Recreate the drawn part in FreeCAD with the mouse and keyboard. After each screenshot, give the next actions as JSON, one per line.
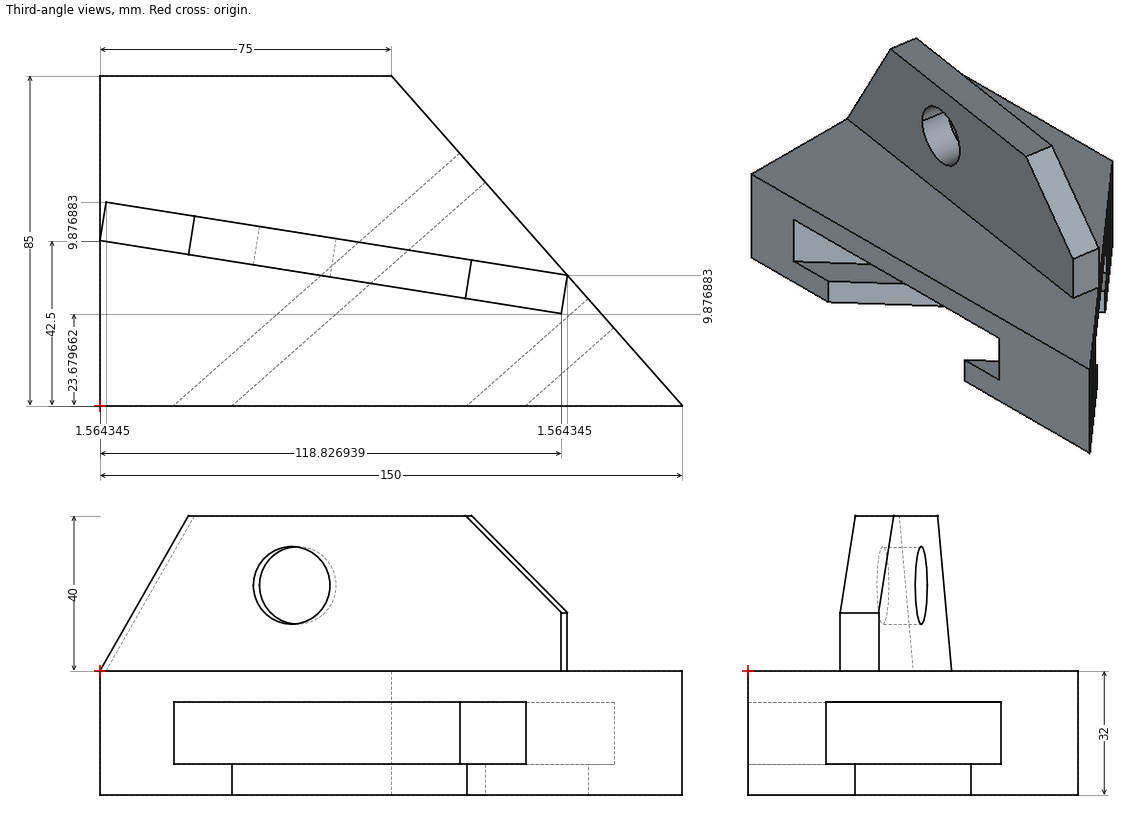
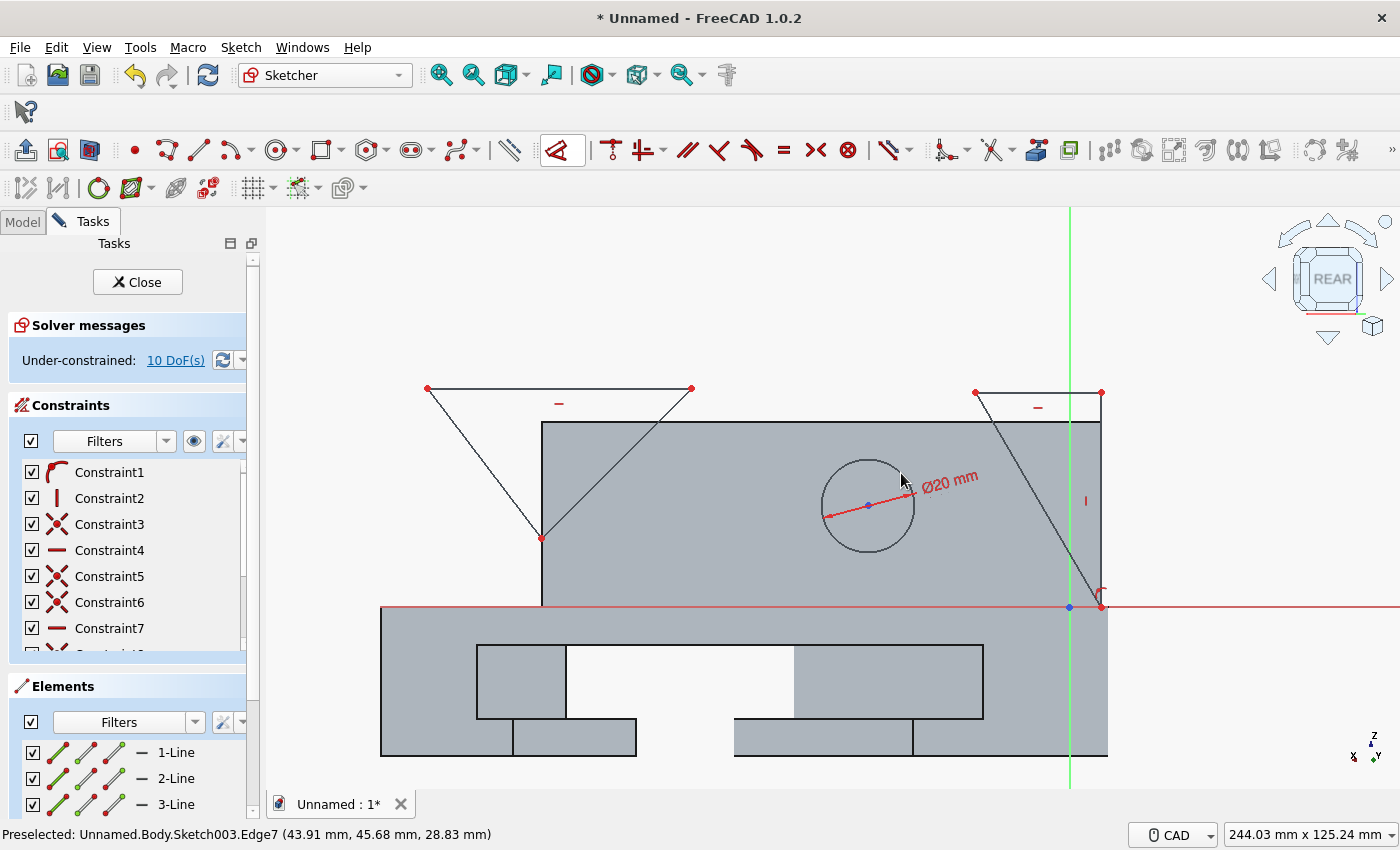
{"action": "left_click", "coordinate": [868, 506]}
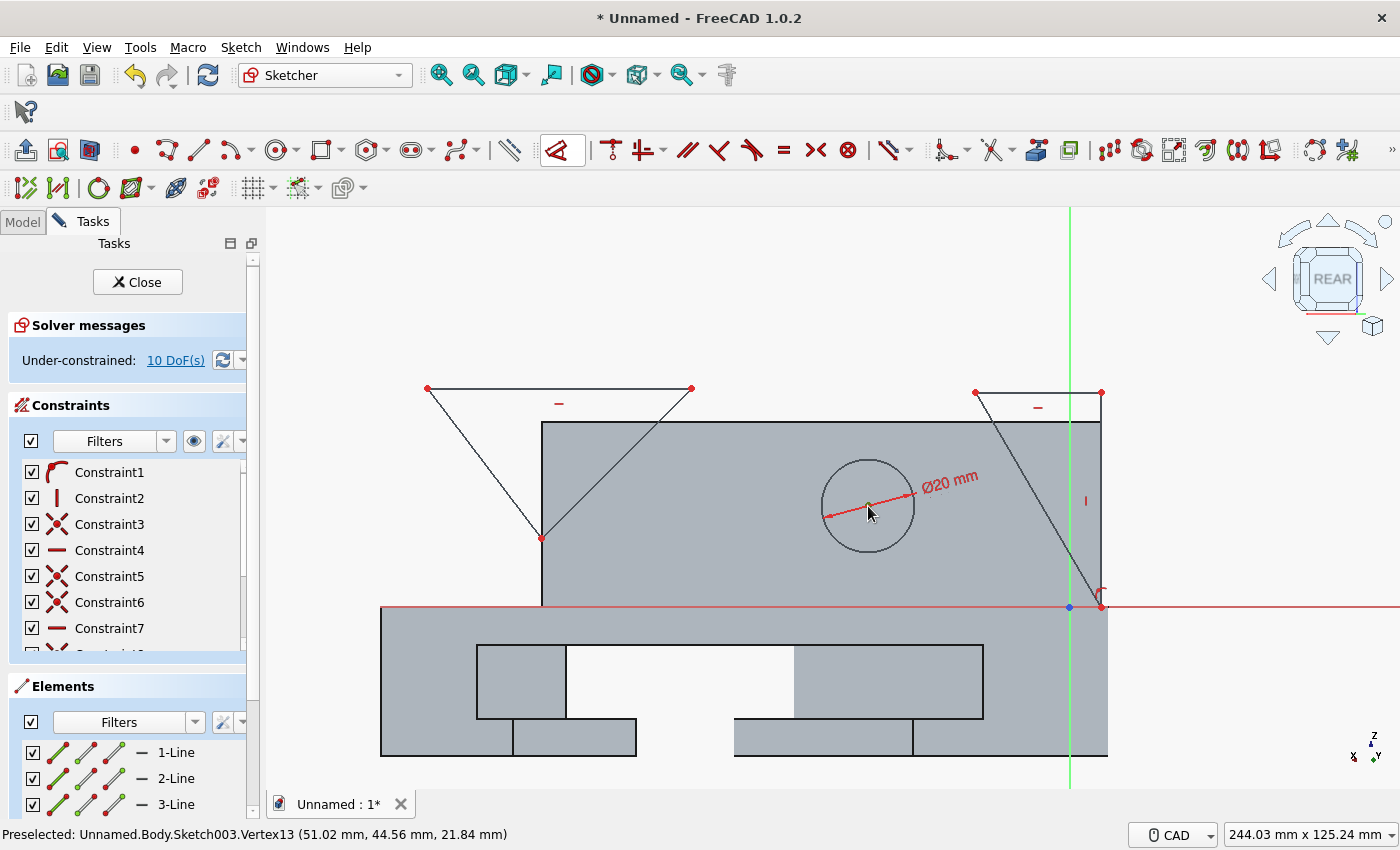
{"action": "left_click", "coordinate": [580, 150]}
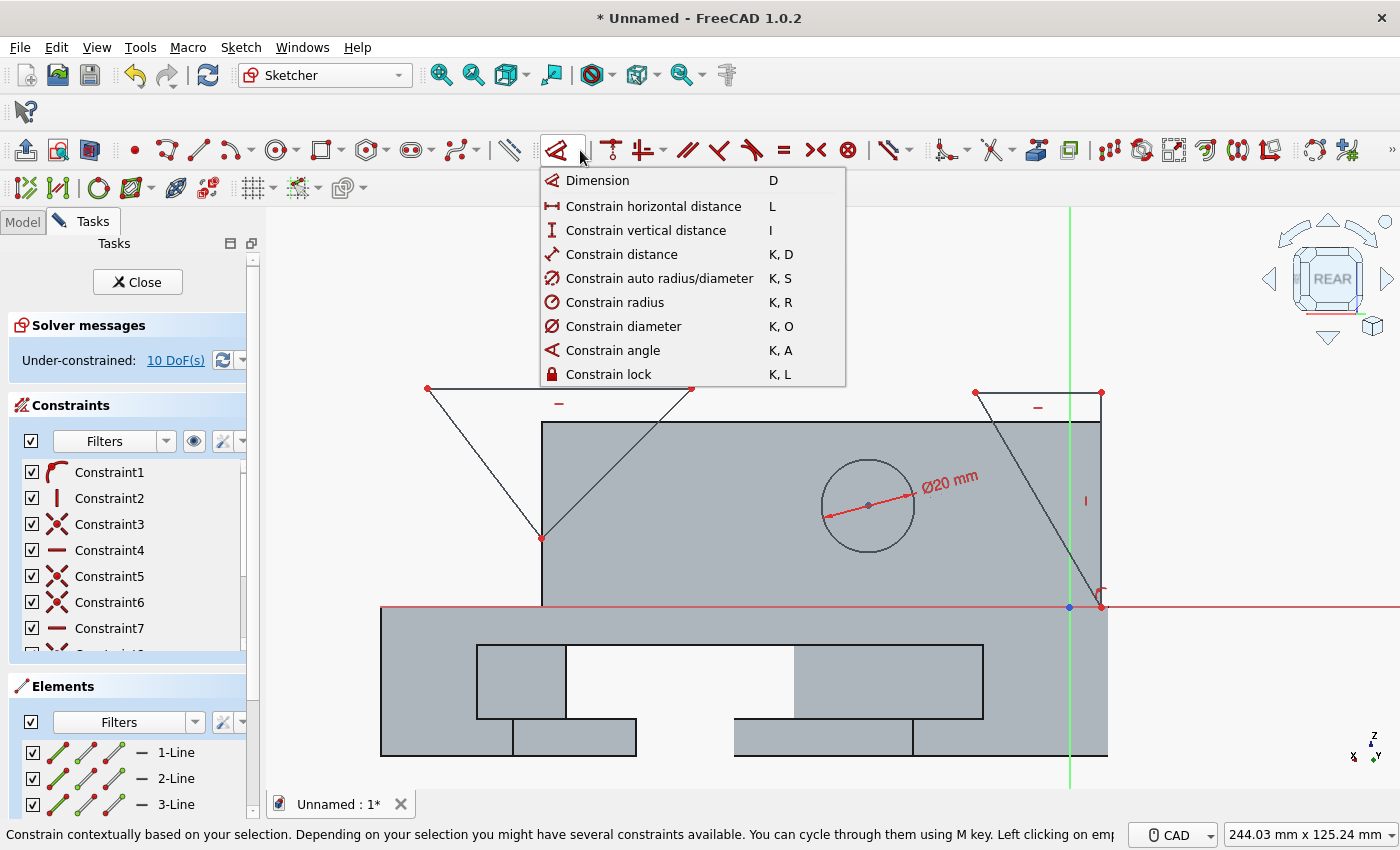
{"action": "left_click", "coordinate": [693, 230]}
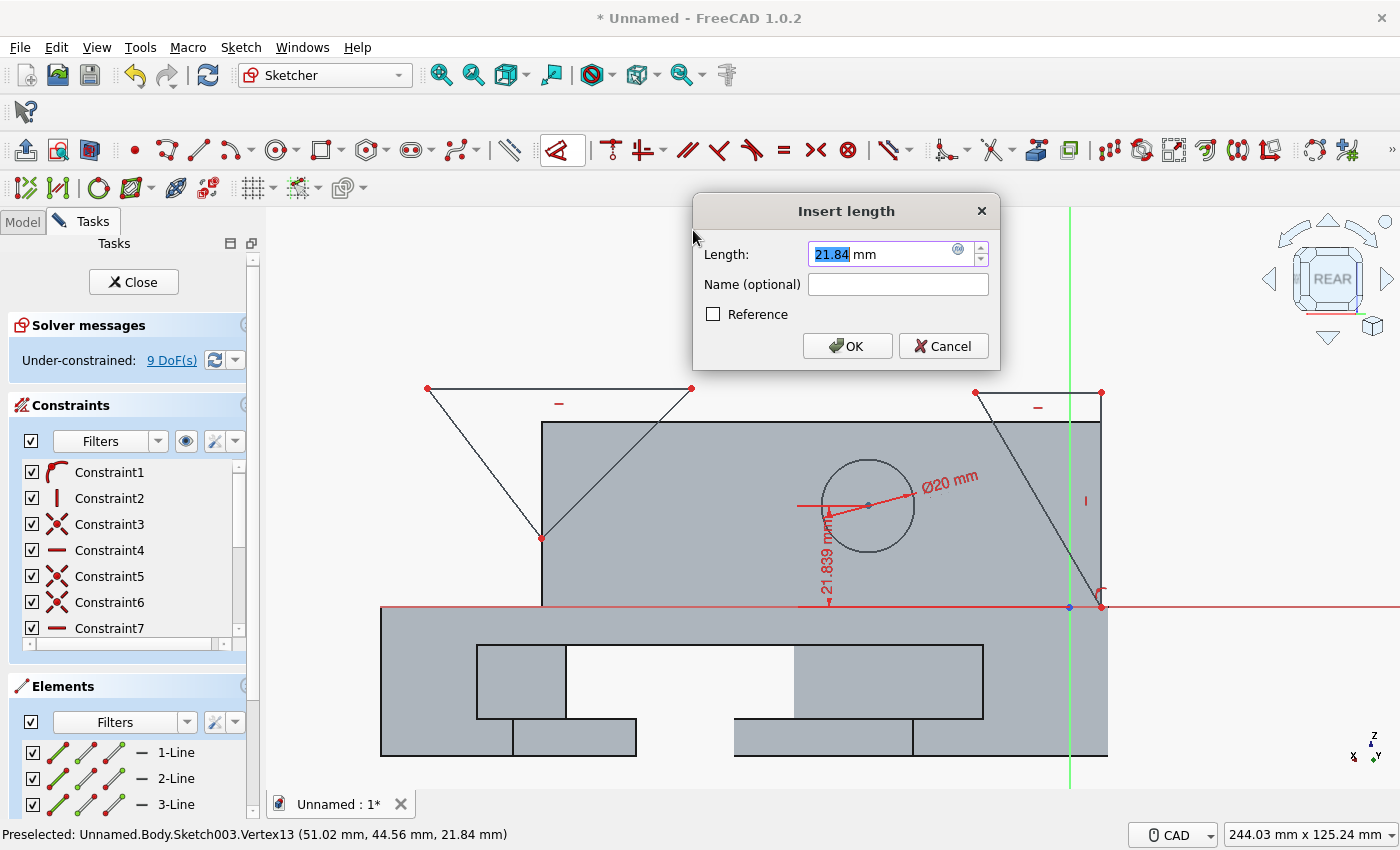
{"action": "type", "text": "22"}
{"action": "key", "text": "Return"}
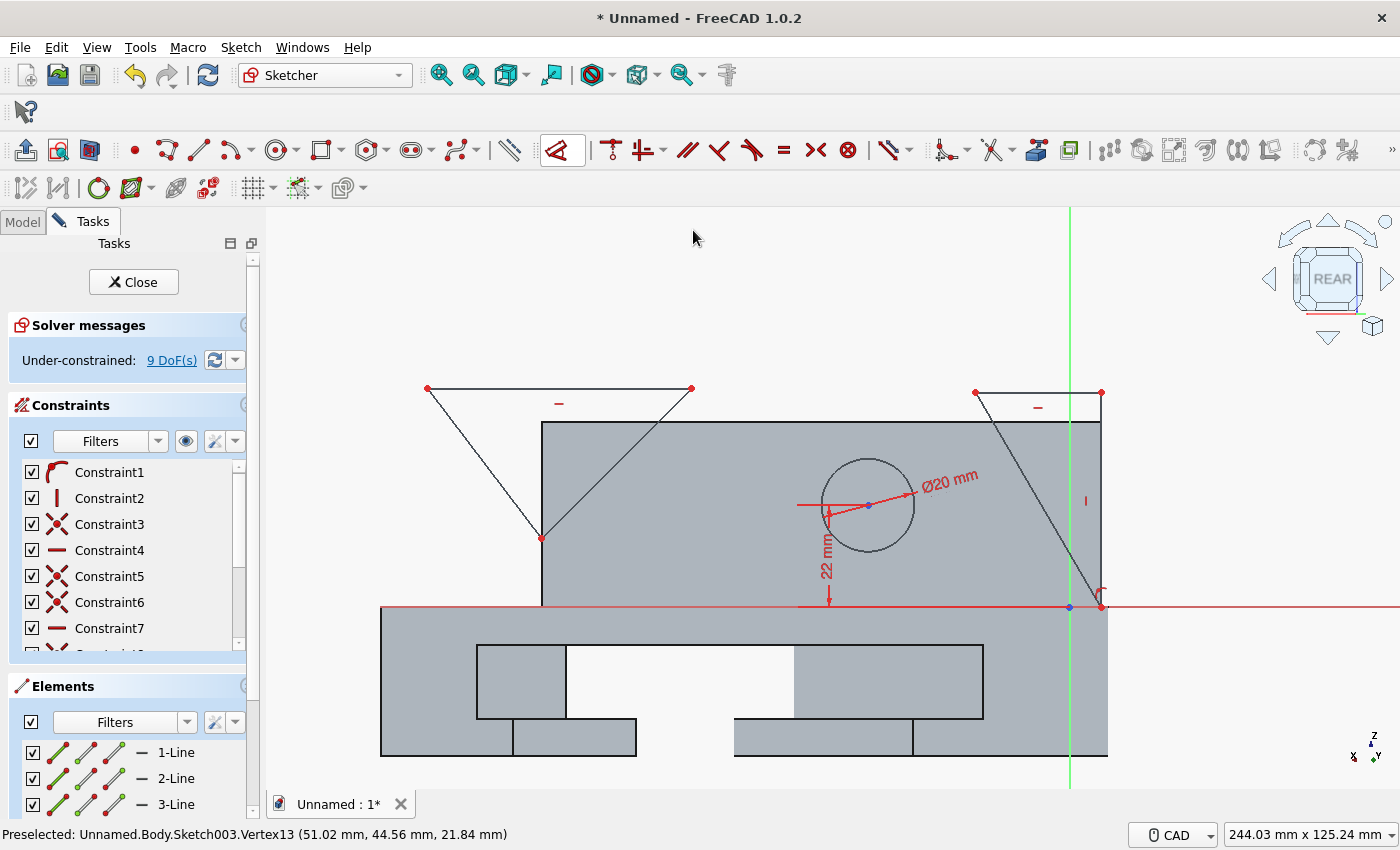
{"action": "left_click", "coordinate": [542, 539]}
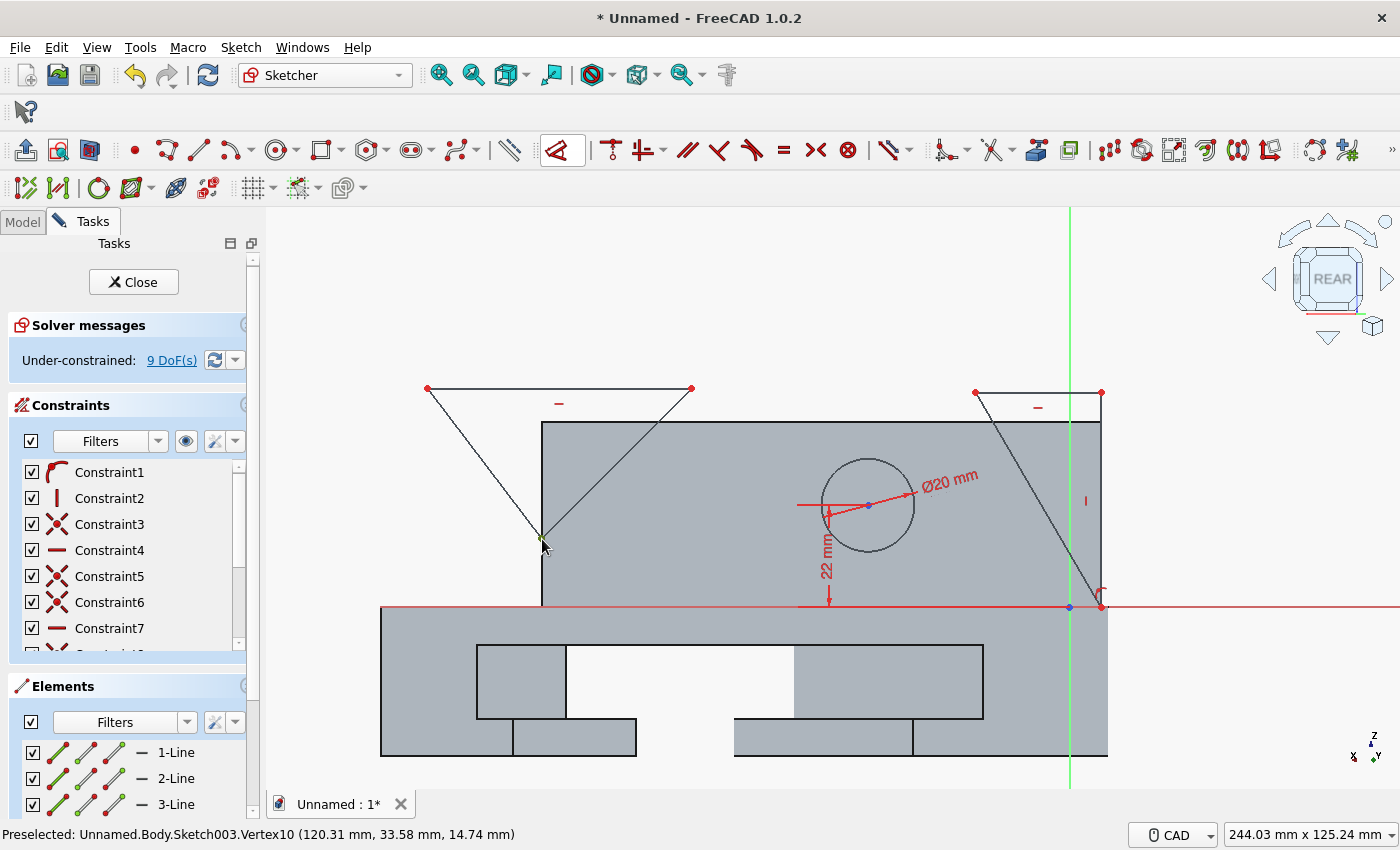
{"action": "left_click", "coordinate": [580, 150]}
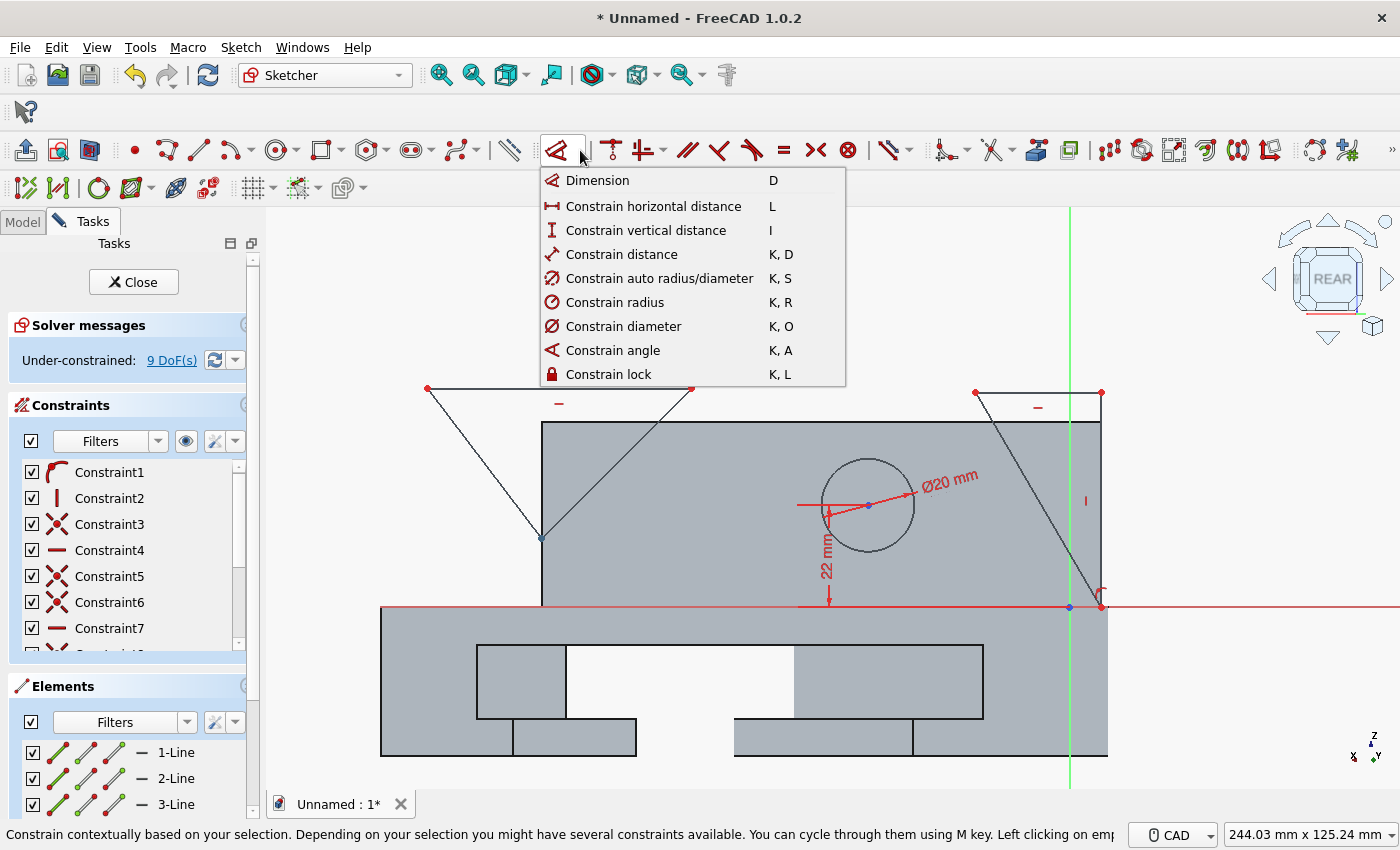
{"action": "left_click", "coordinate": [693, 230]}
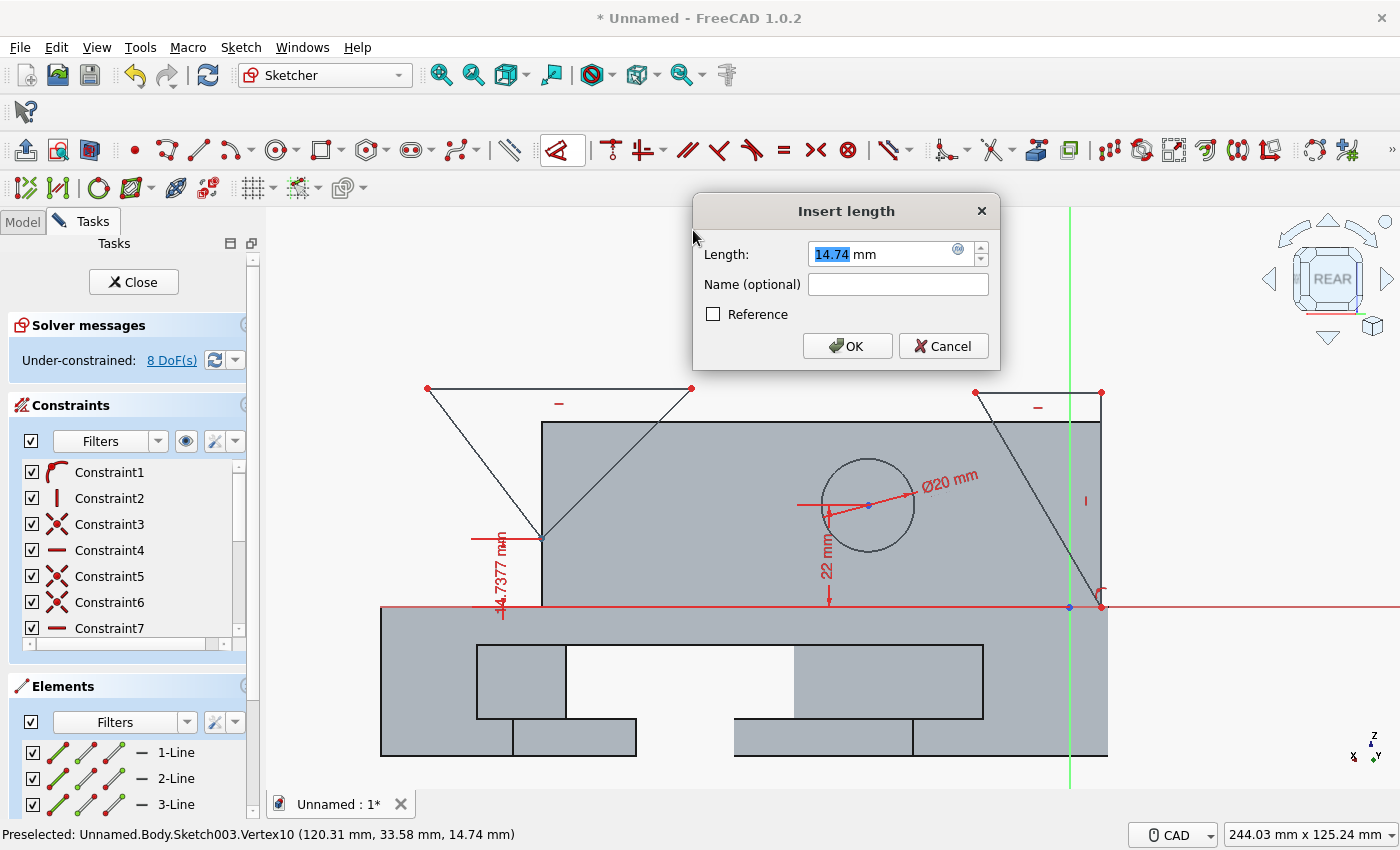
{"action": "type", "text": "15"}
{"action": "key", "text": "Return"}